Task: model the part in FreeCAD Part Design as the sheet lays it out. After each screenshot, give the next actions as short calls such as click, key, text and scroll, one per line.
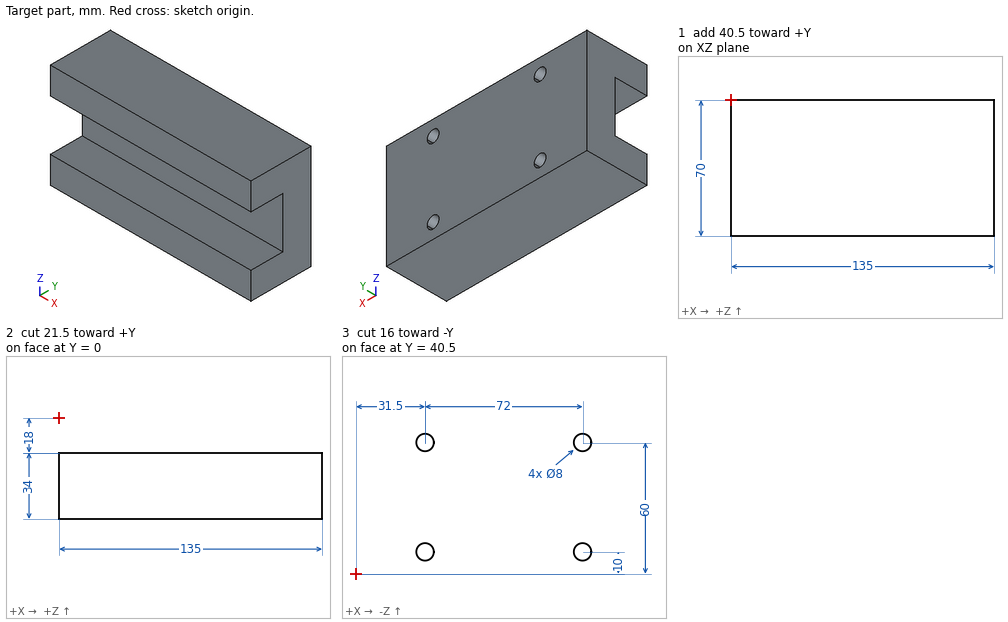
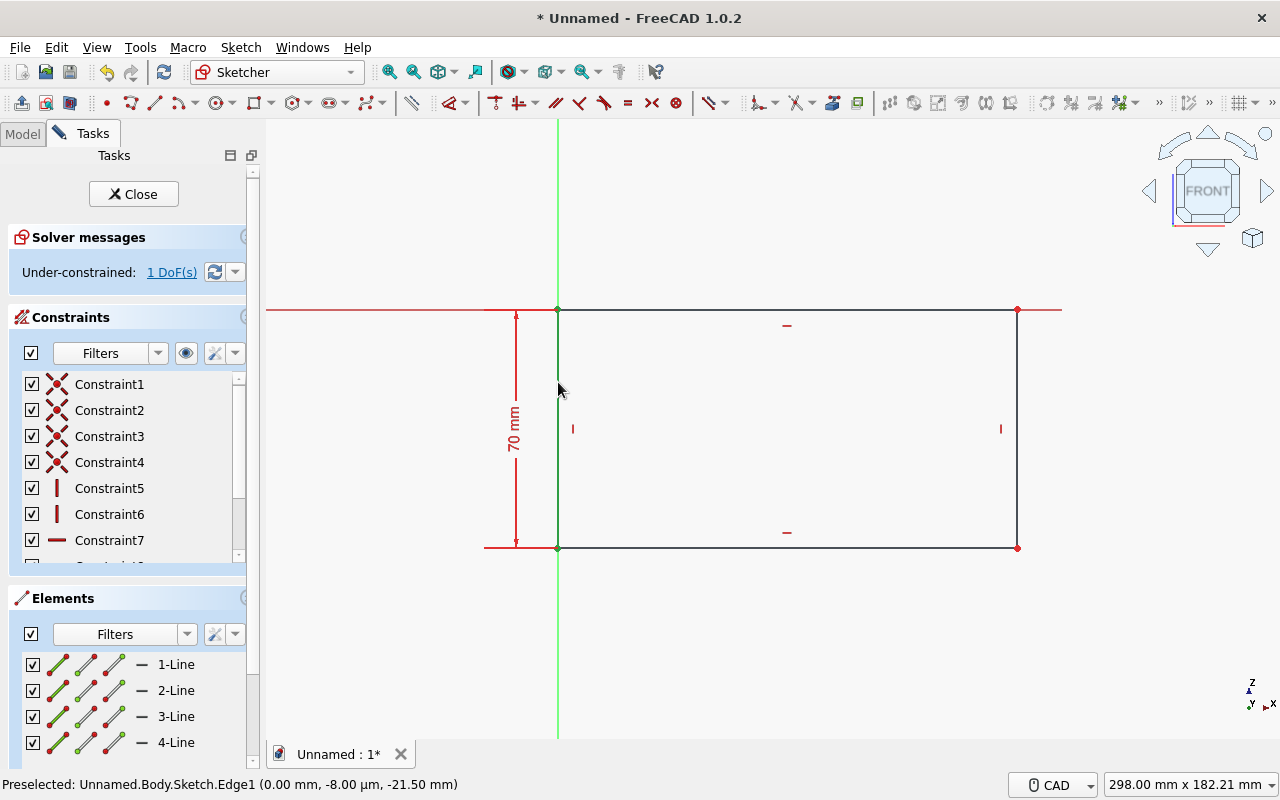
click(695, 548)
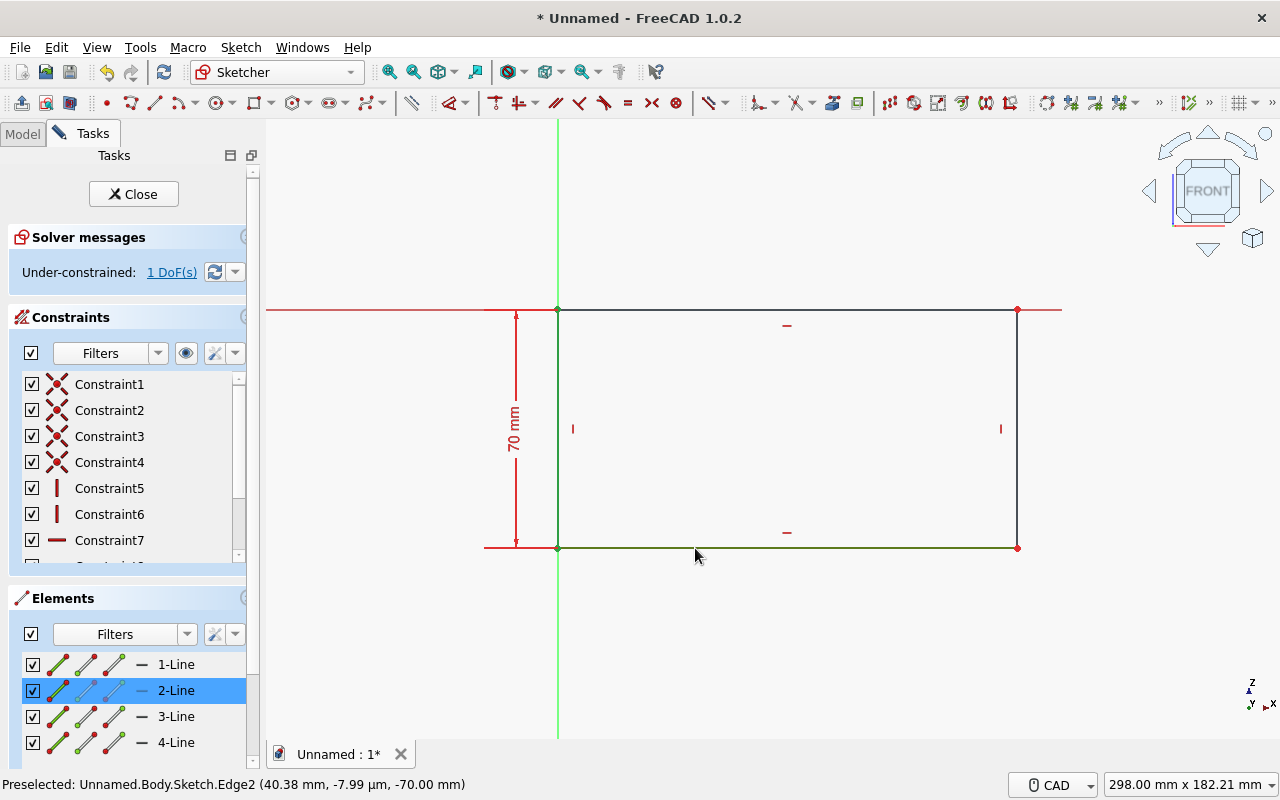
key(l)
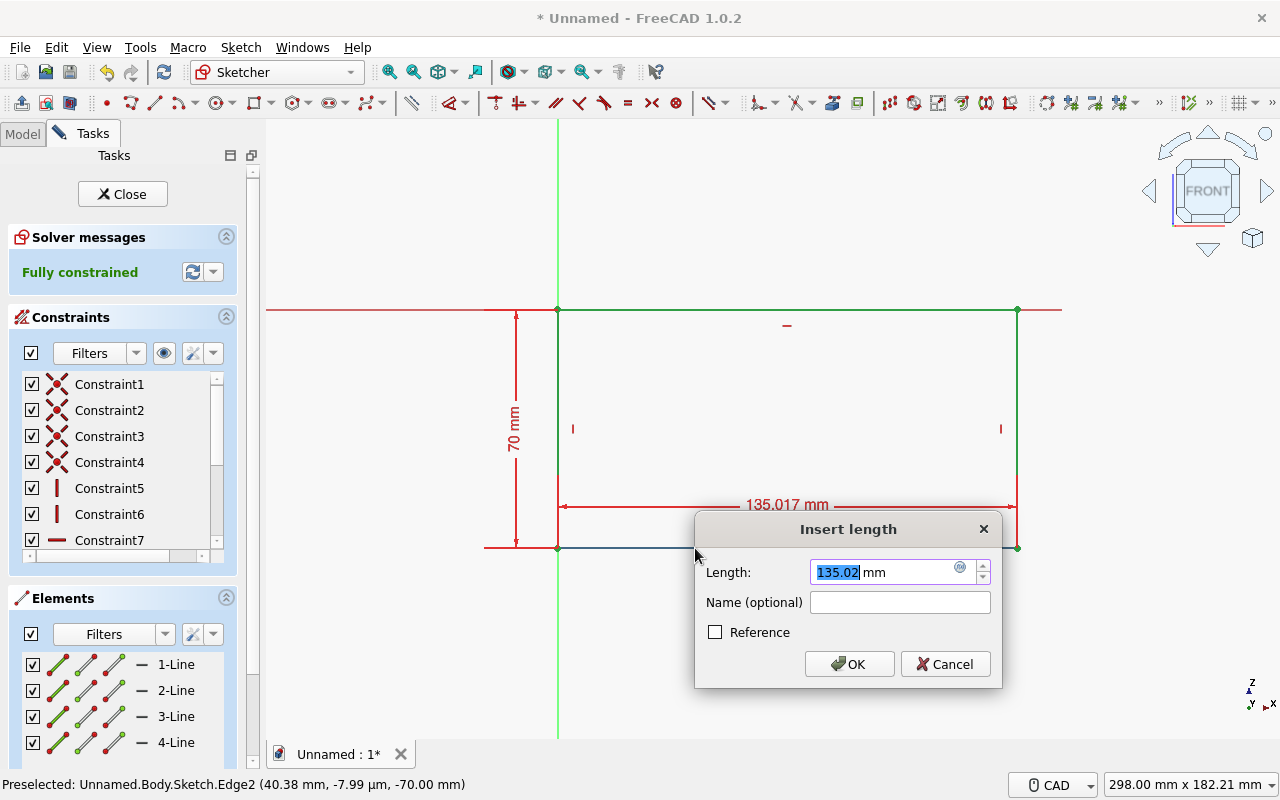
text(135)
key(Return)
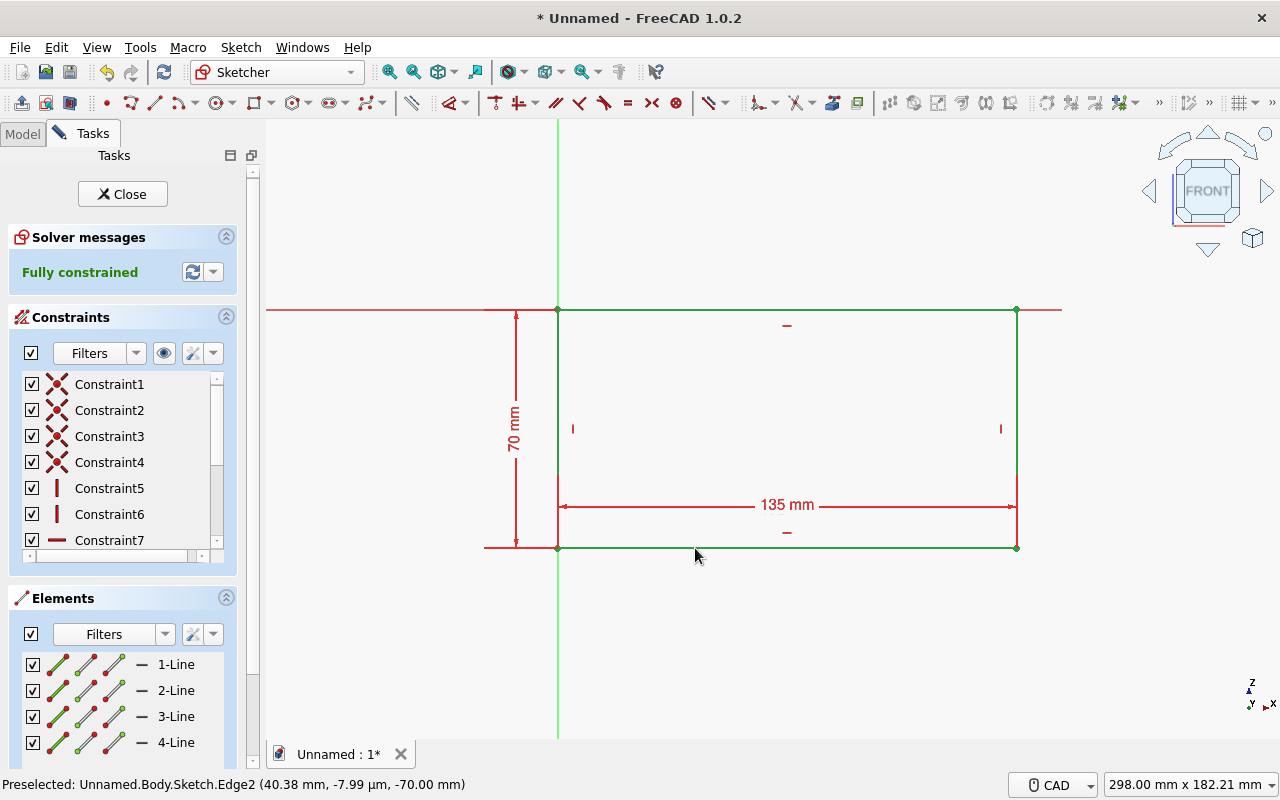
click(123, 194)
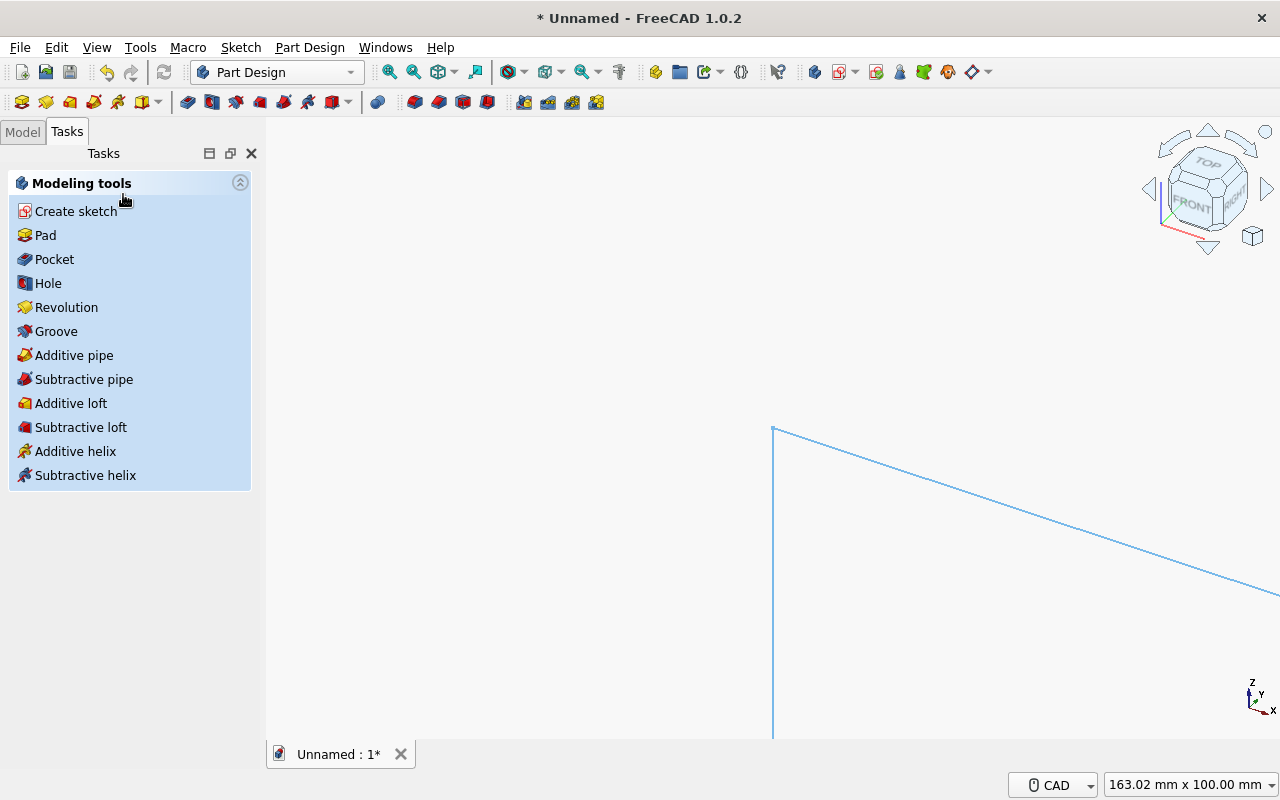
click(22, 102)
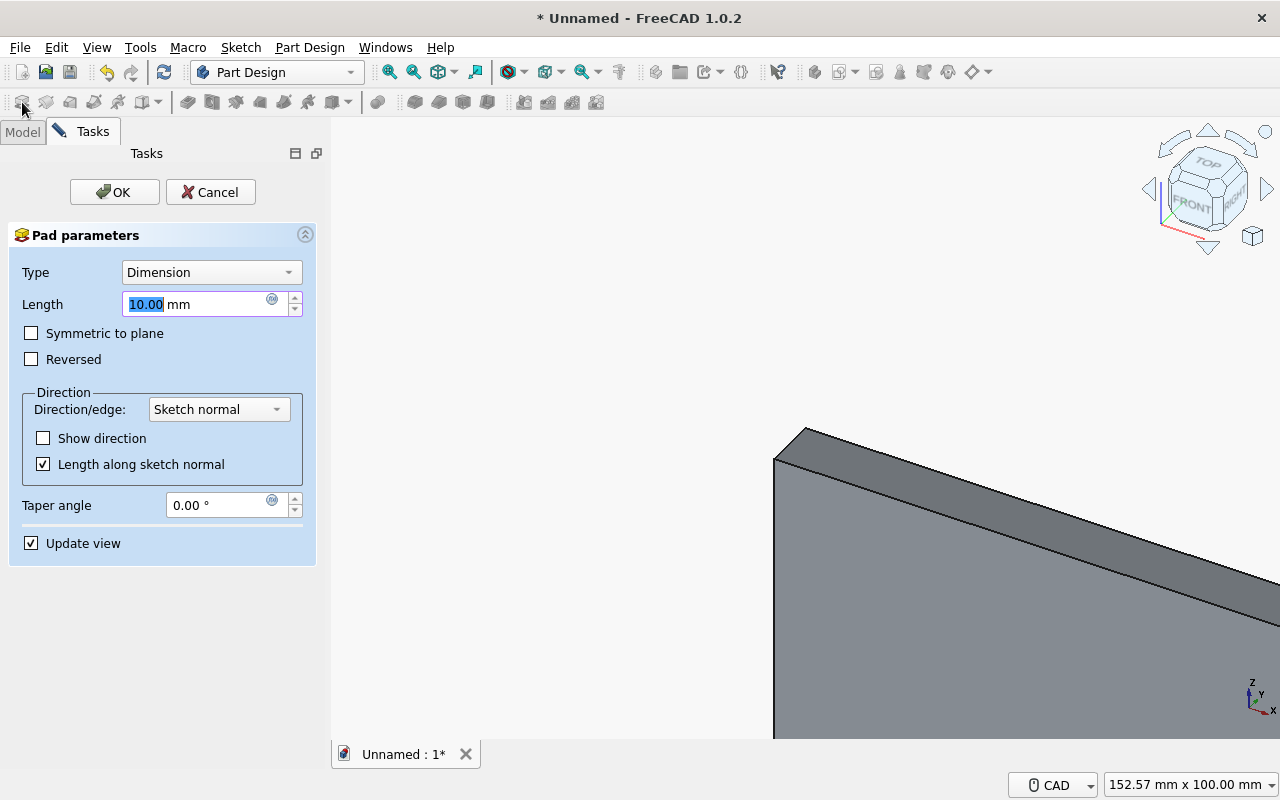
text(40.5)
key(Tab)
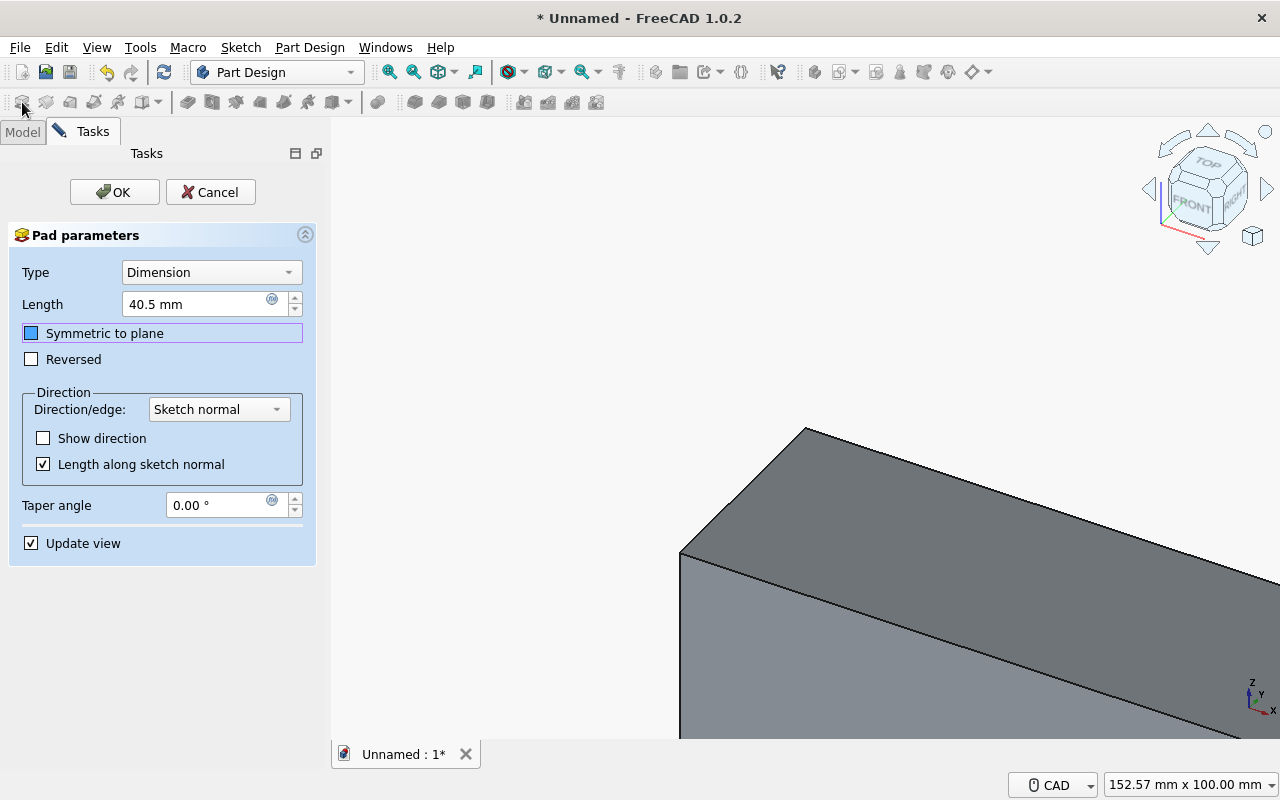
click(30, 359)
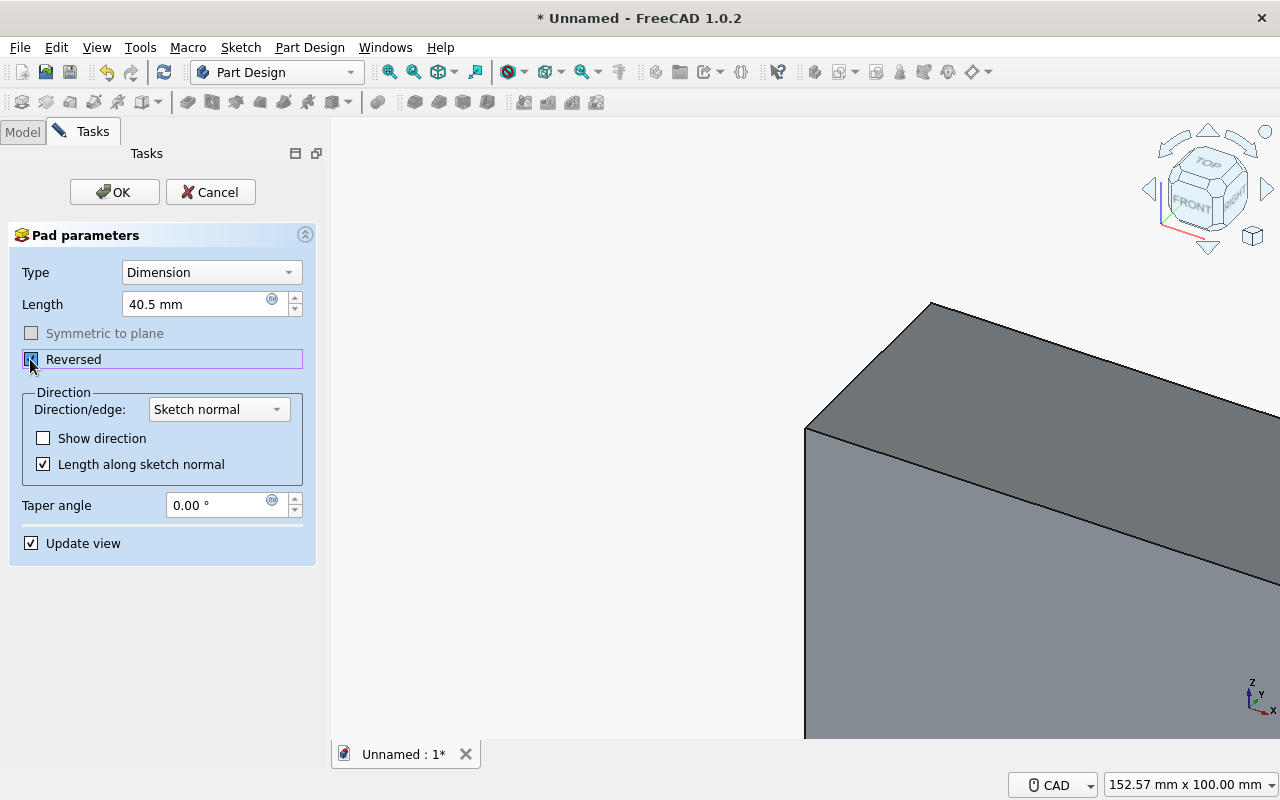
click(115, 192)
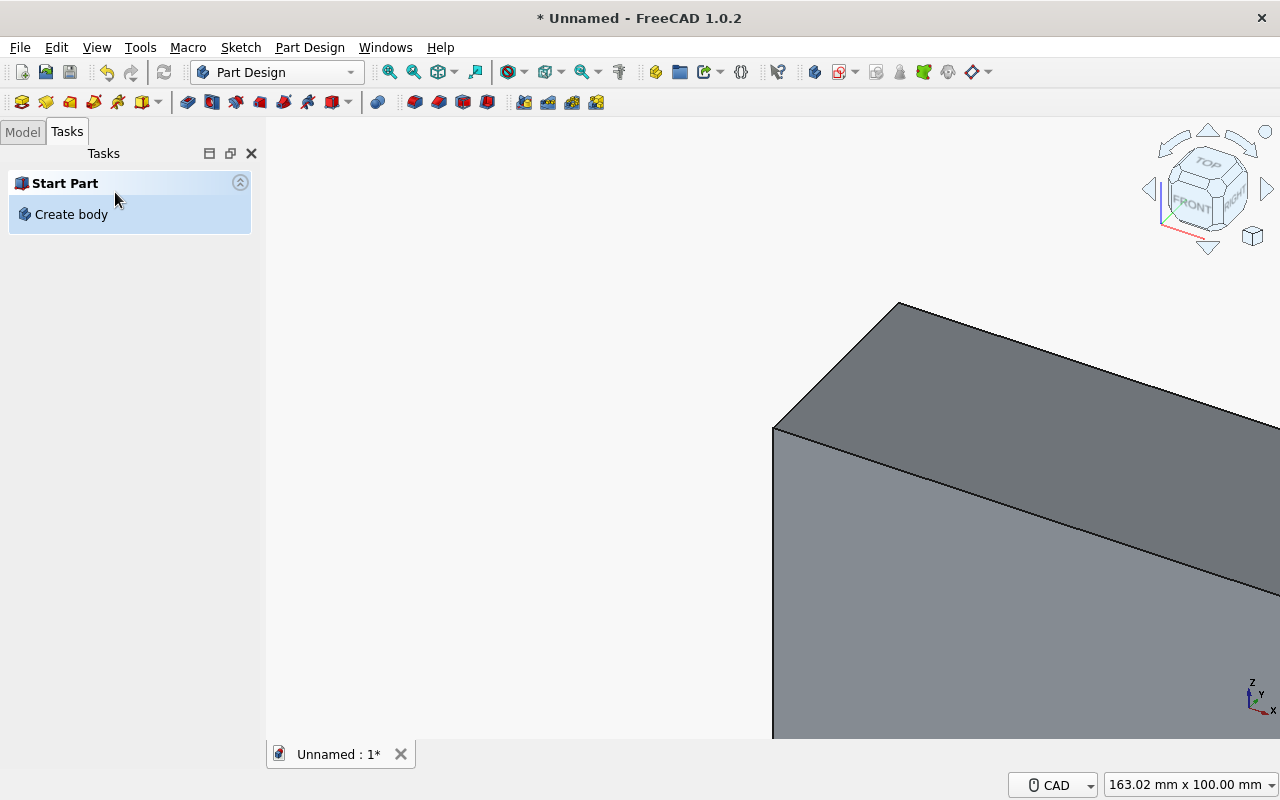
click(390, 72)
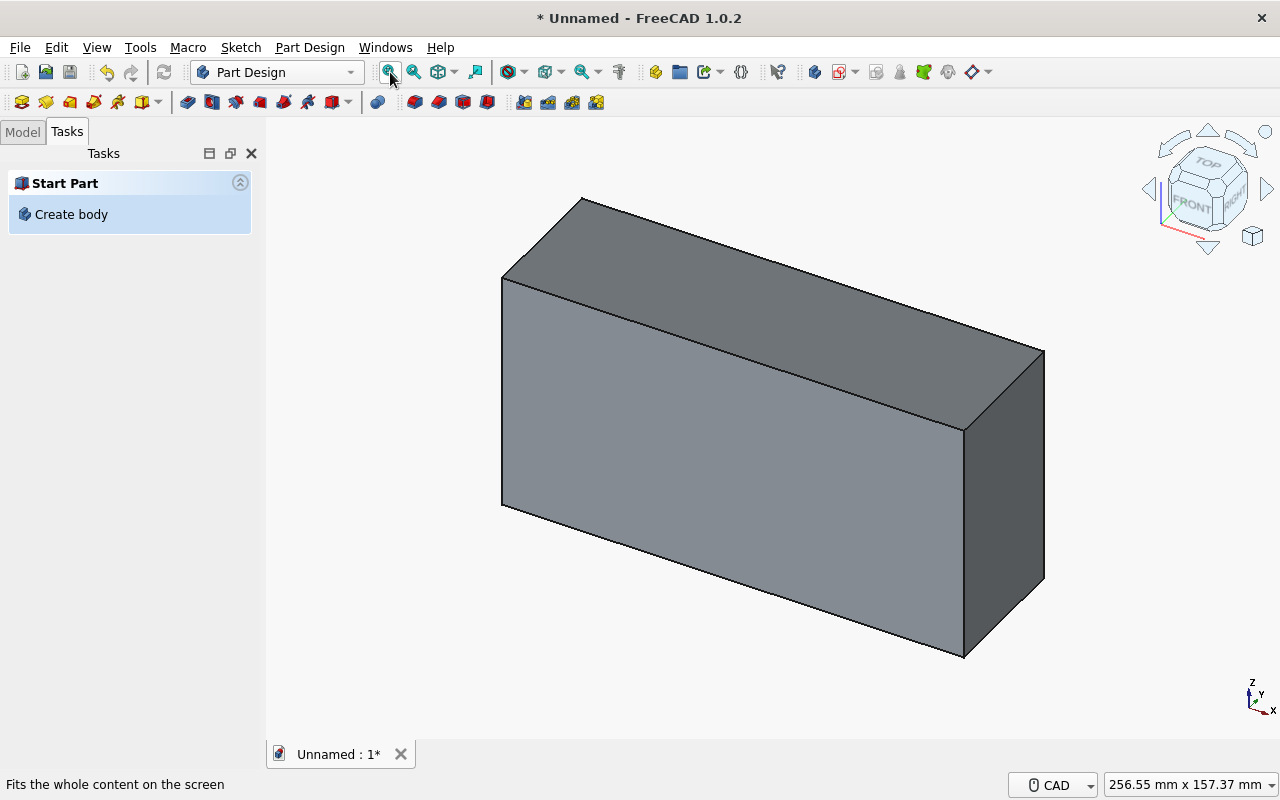
click(799, 489)